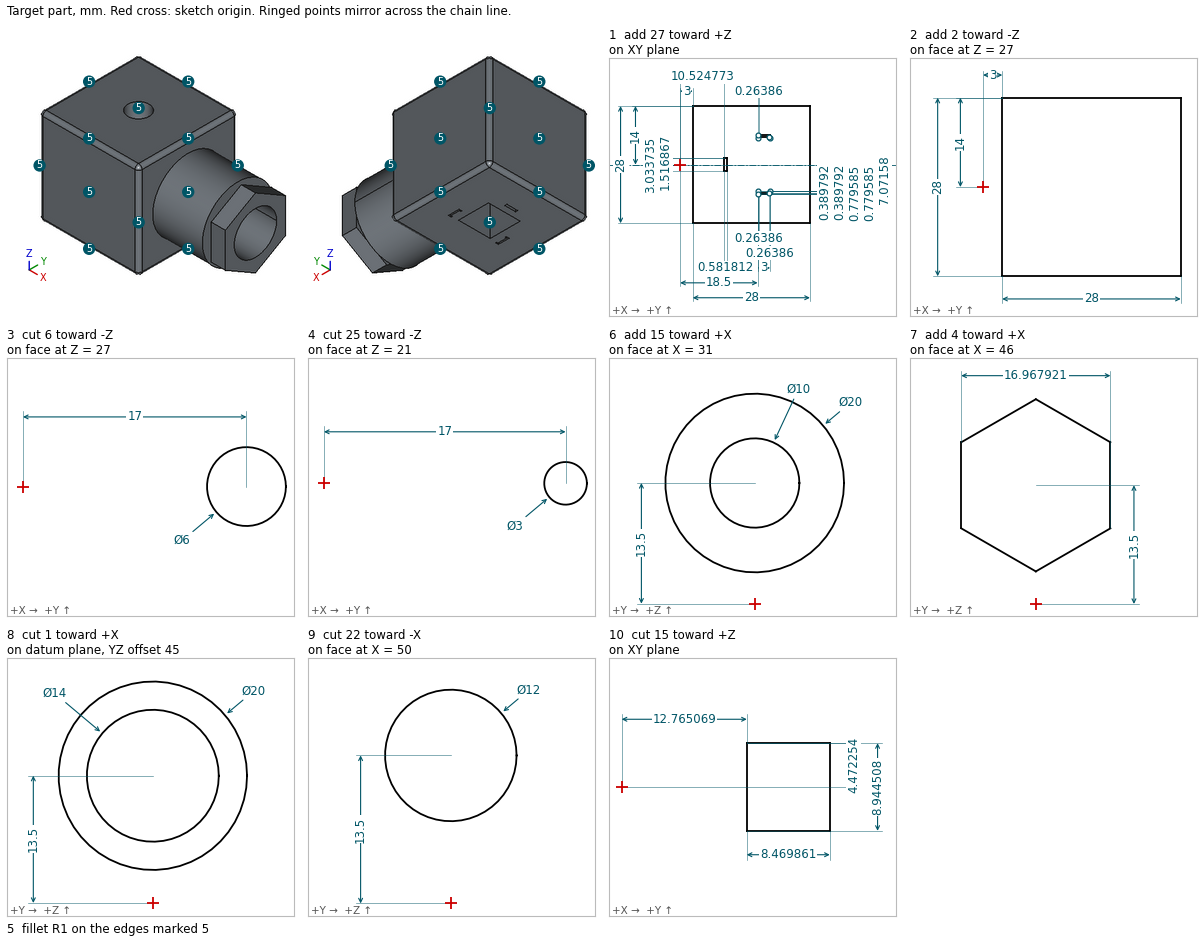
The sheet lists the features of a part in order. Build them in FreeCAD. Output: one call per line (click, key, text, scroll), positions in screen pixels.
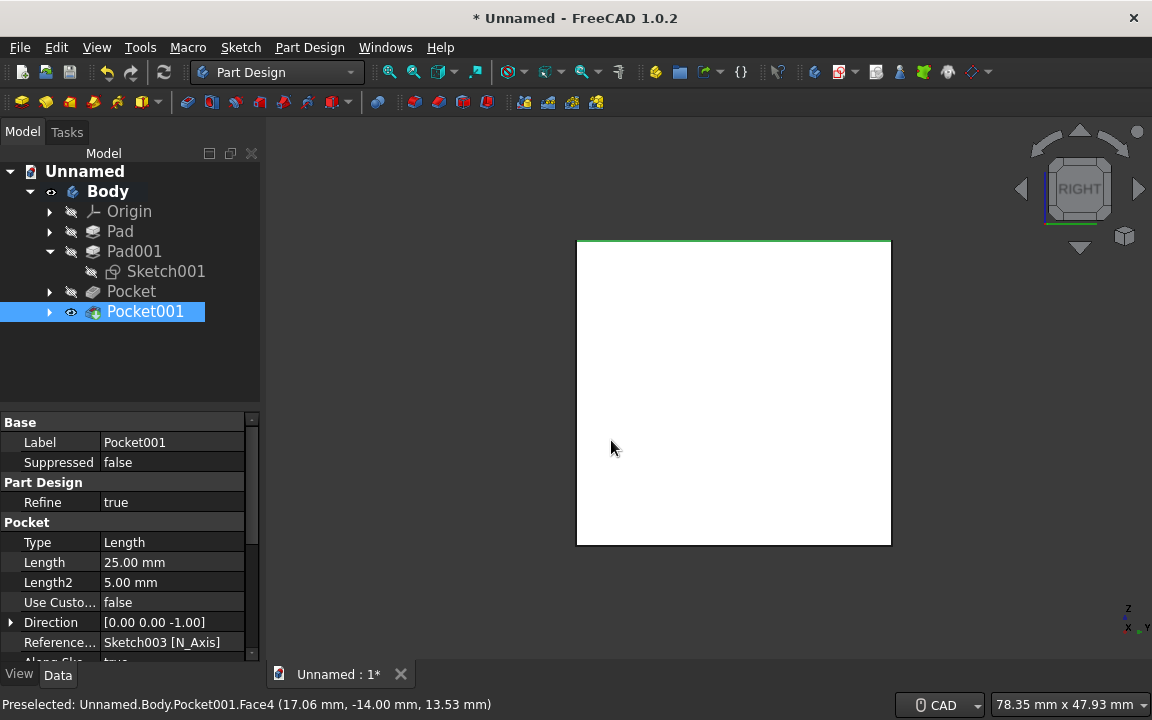
click(734, 545, ctrl)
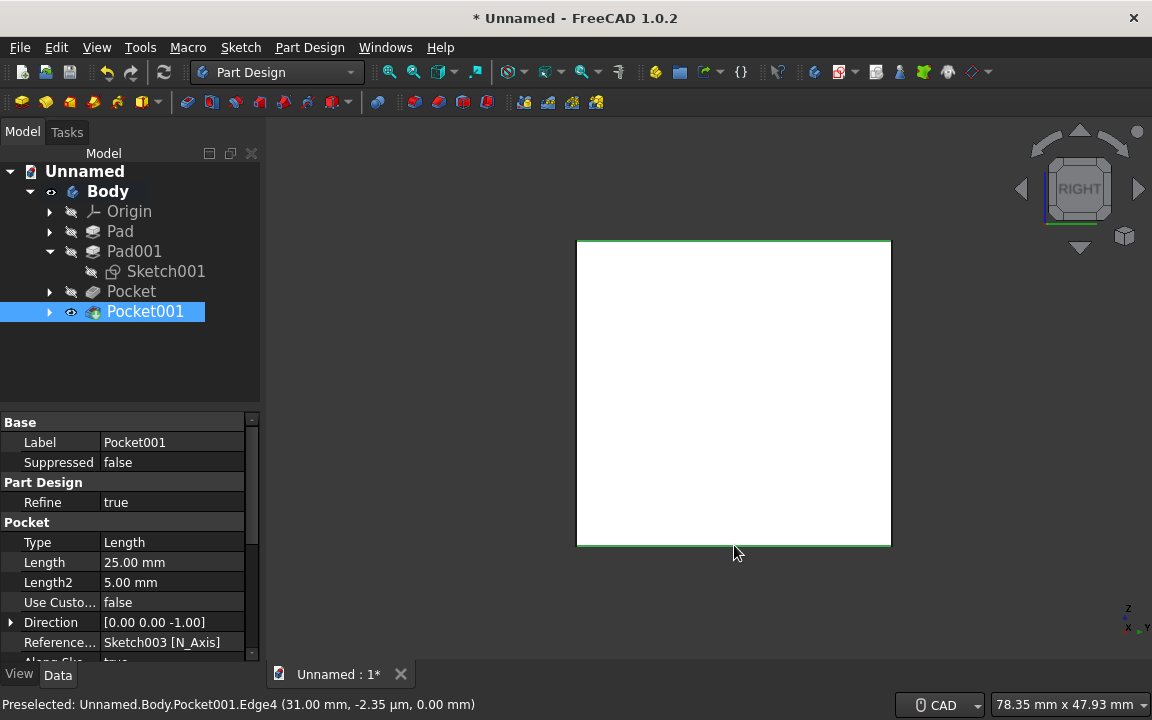
key(5)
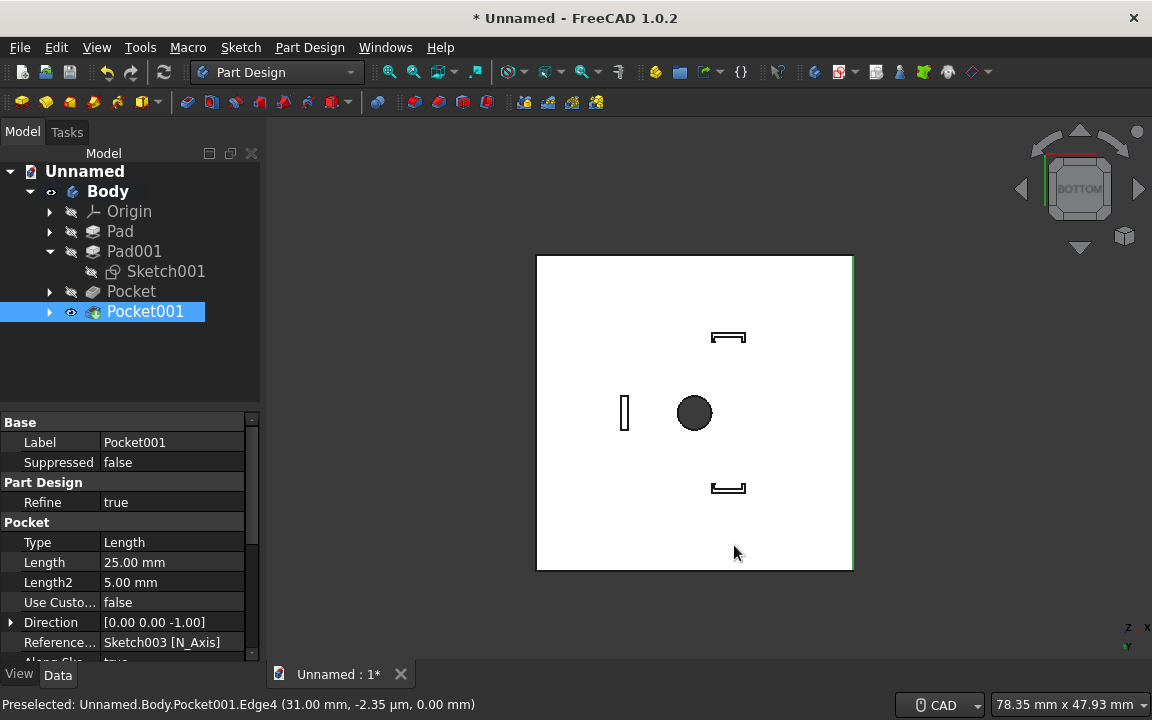
key(4)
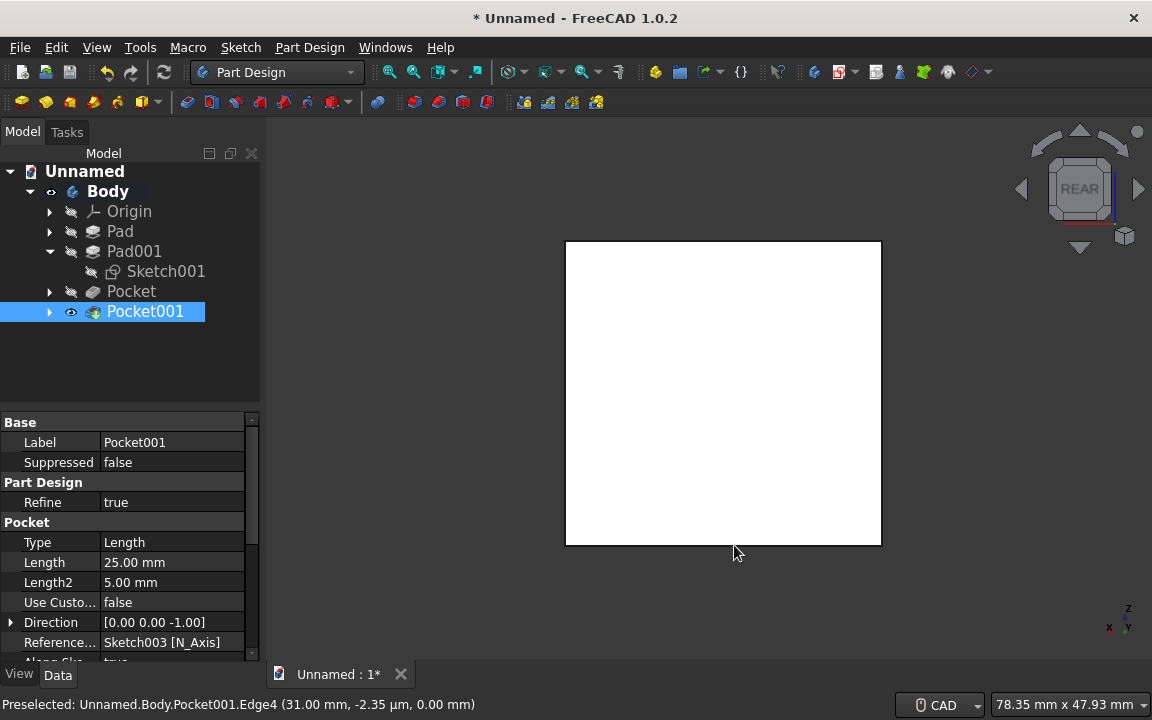
click(723, 392, ctrl)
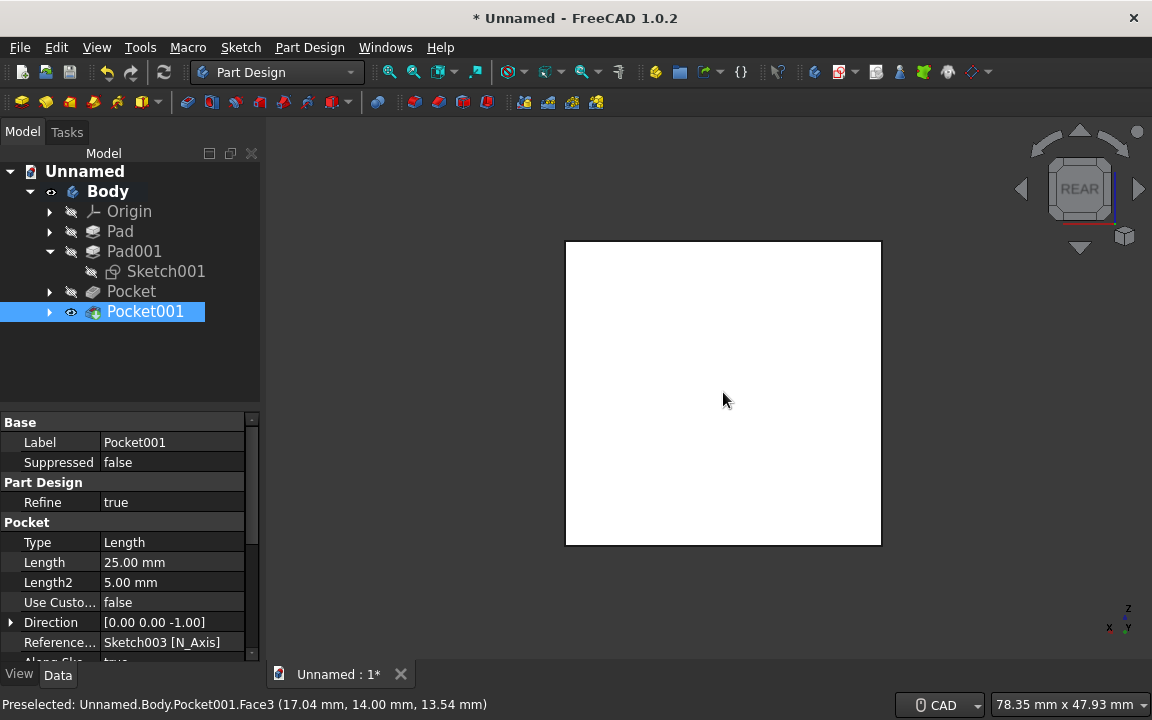
key(6)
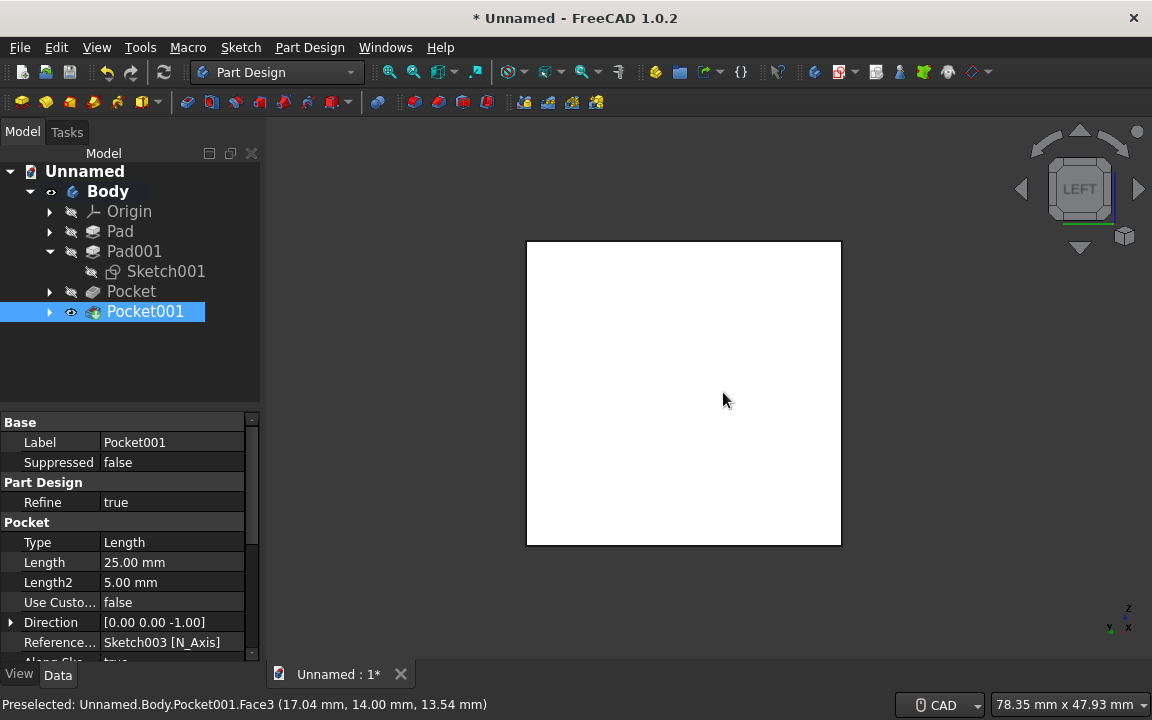
click(684, 392, ctrl)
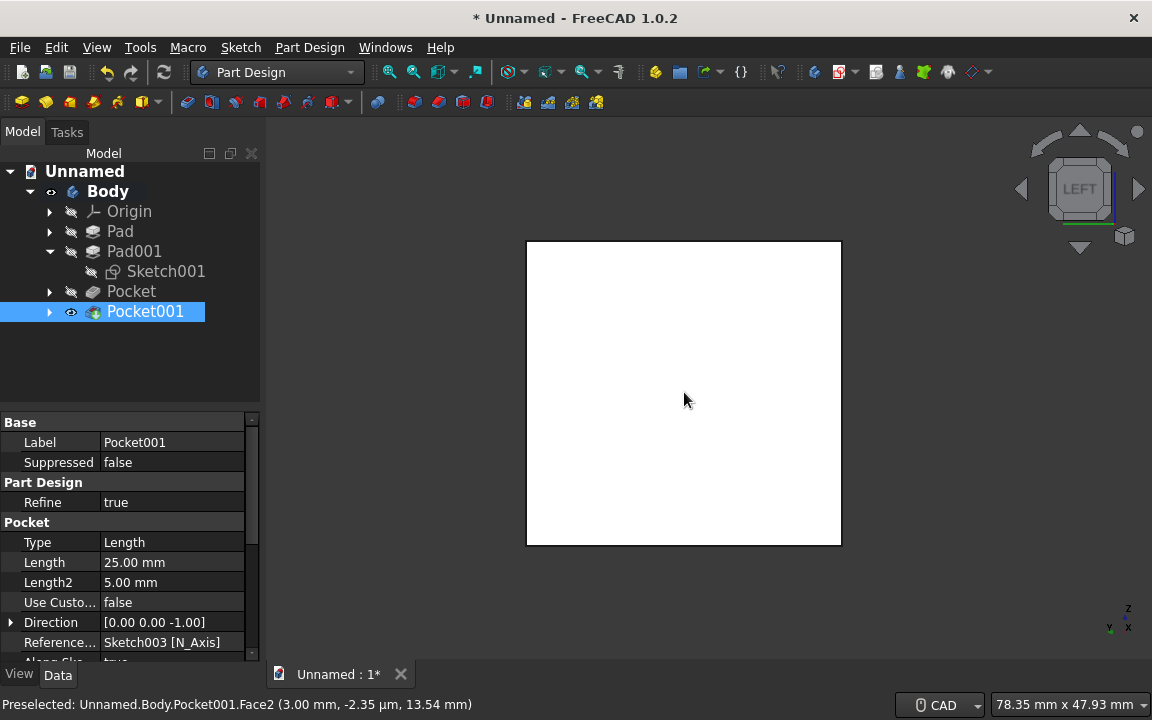
click(416, 102)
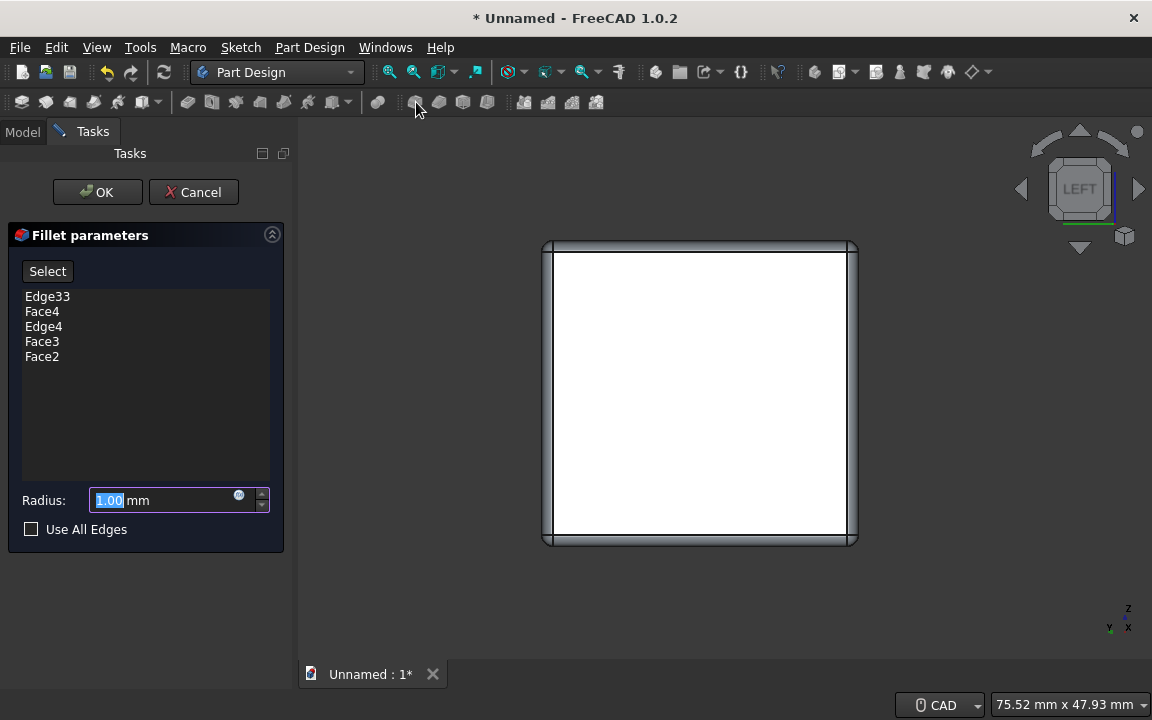
text(1)
key(Tab)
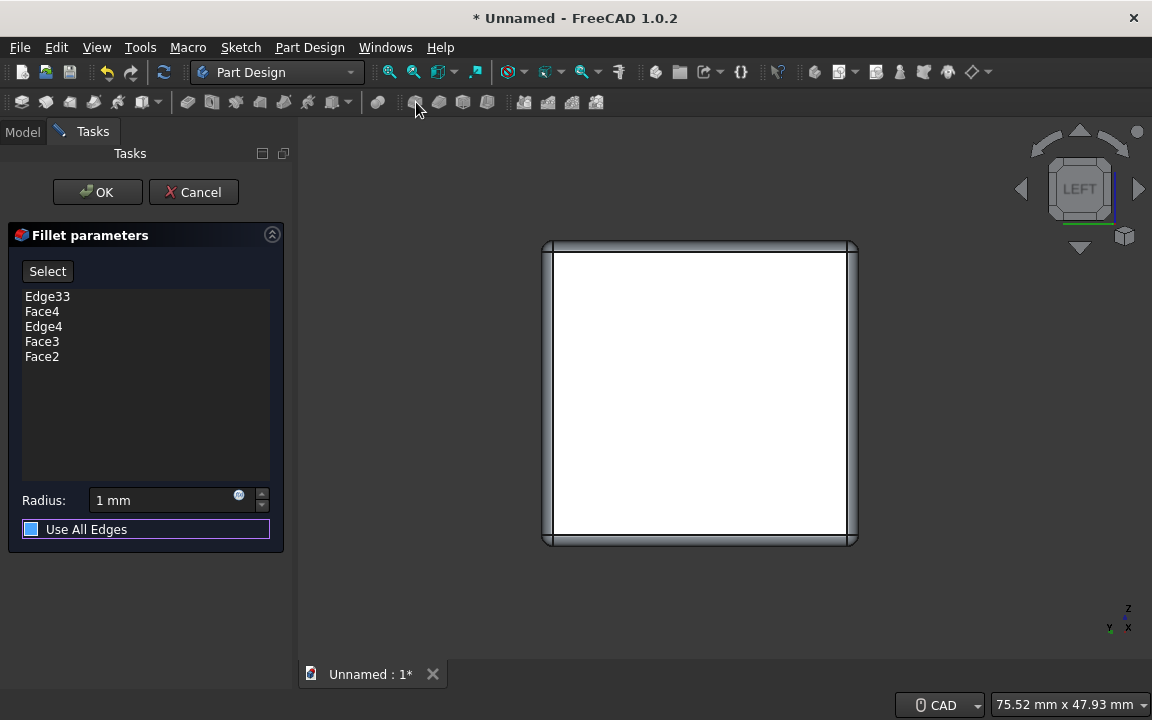
click(98, 192)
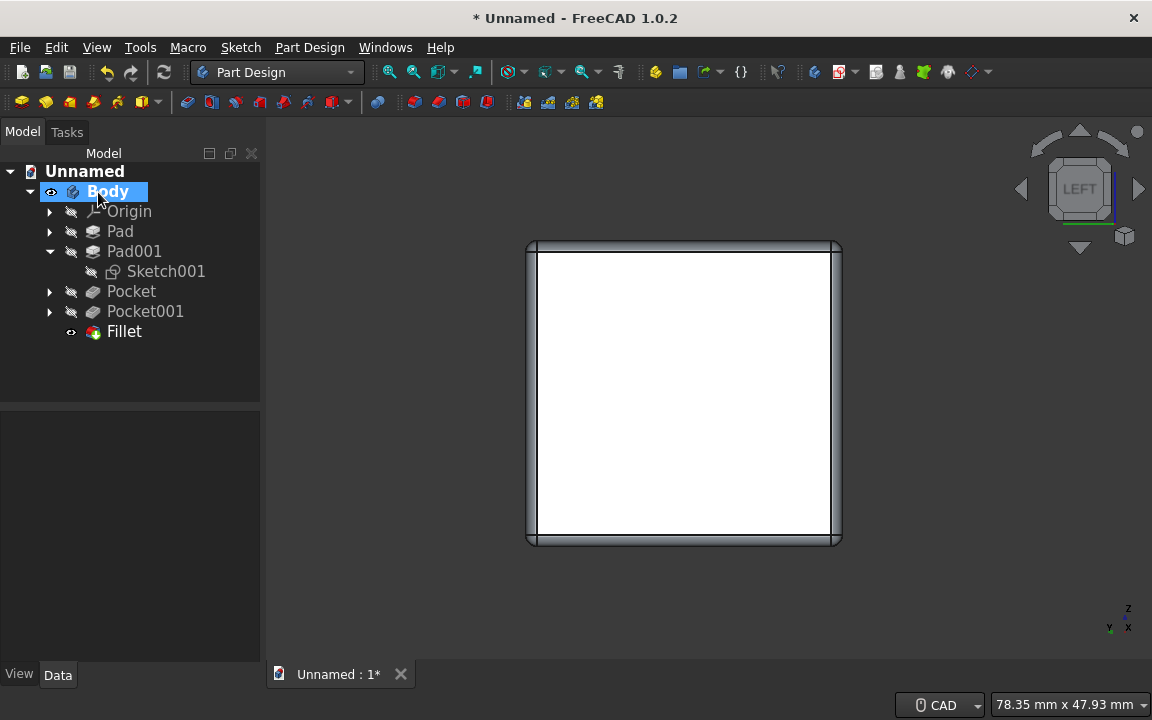
key(0)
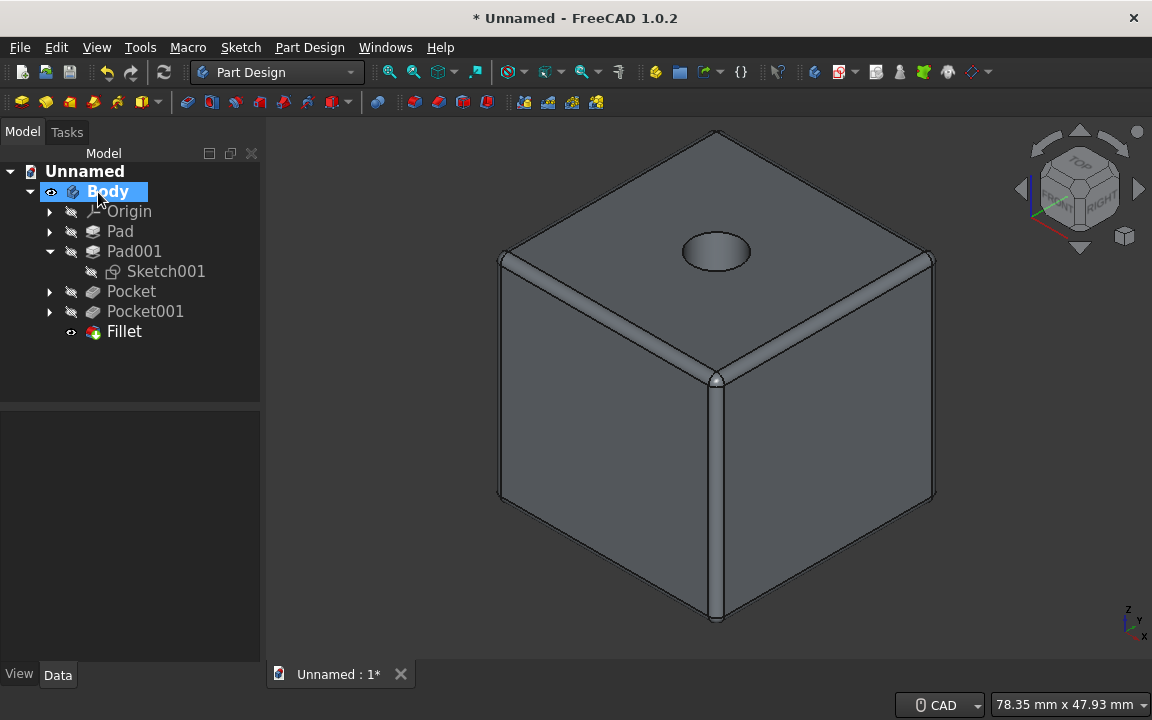
click(828, 440)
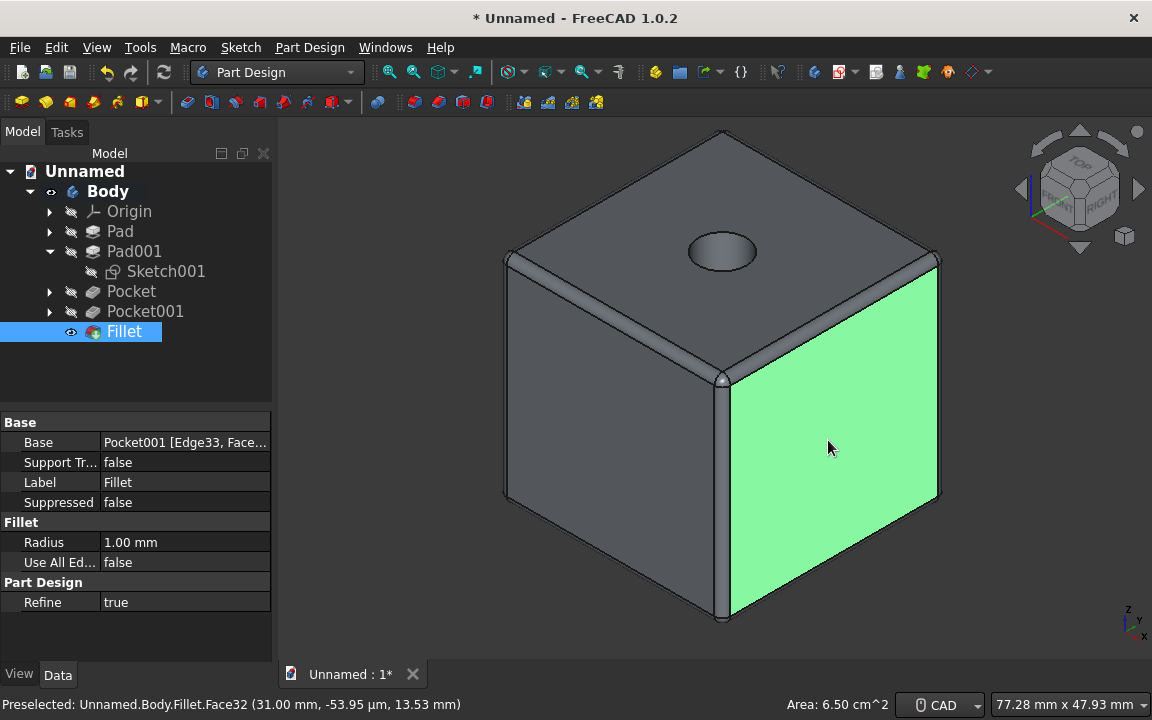
click(840, 72)